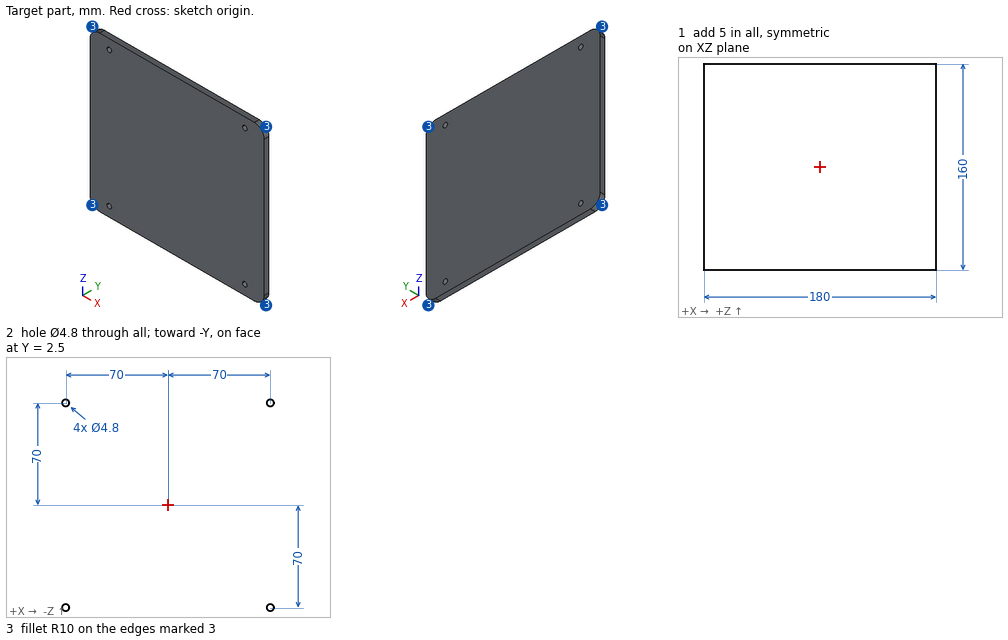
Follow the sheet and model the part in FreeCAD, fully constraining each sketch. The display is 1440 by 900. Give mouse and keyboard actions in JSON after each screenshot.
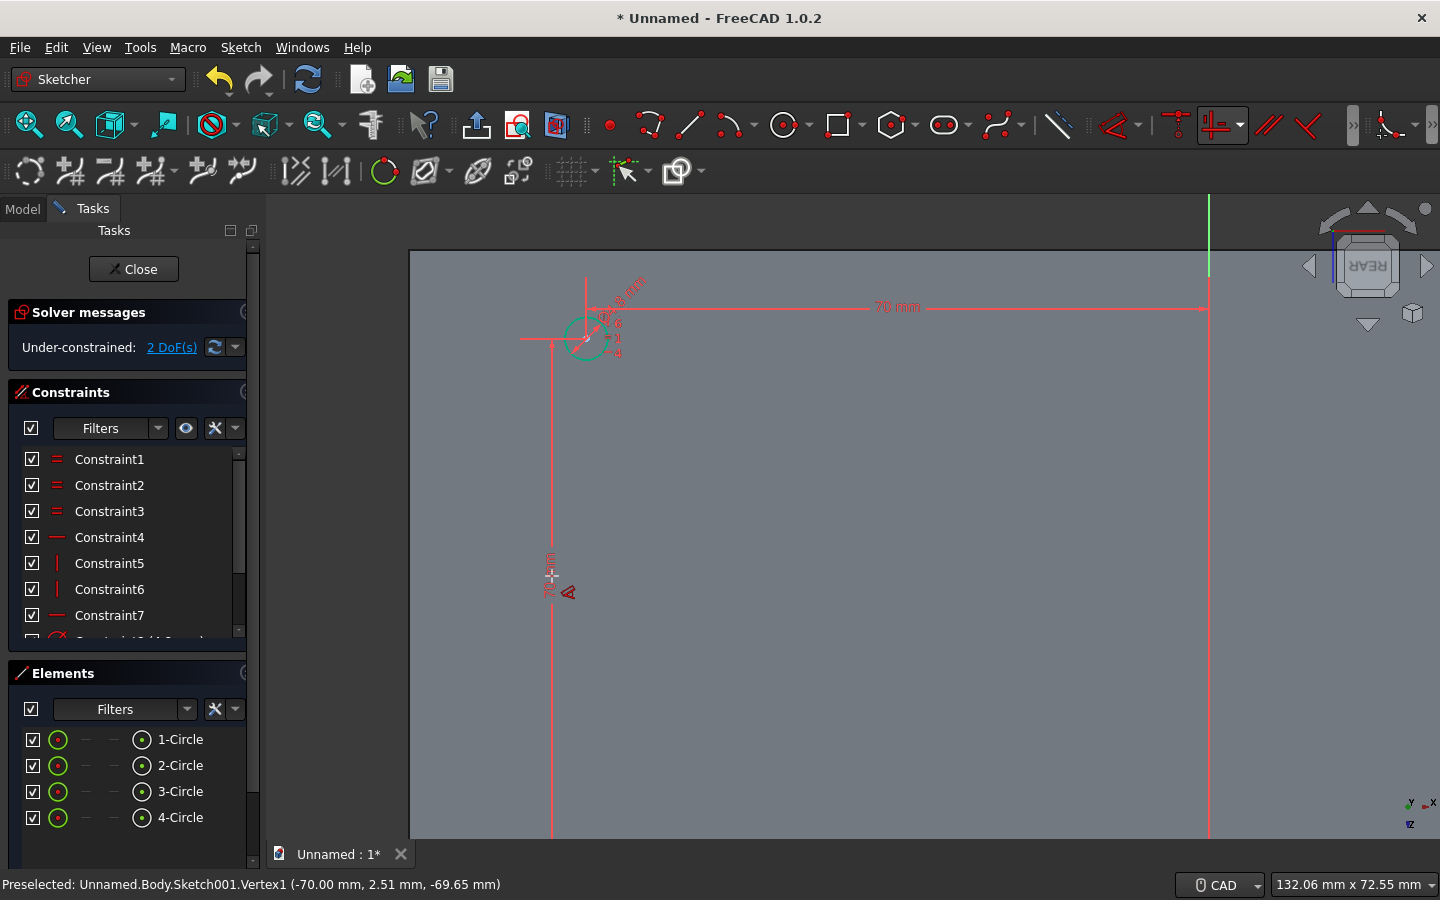
{"action": "scroll", "coordinate": [602, 325], "scroll_direction": "down", "scroll_amount": 6}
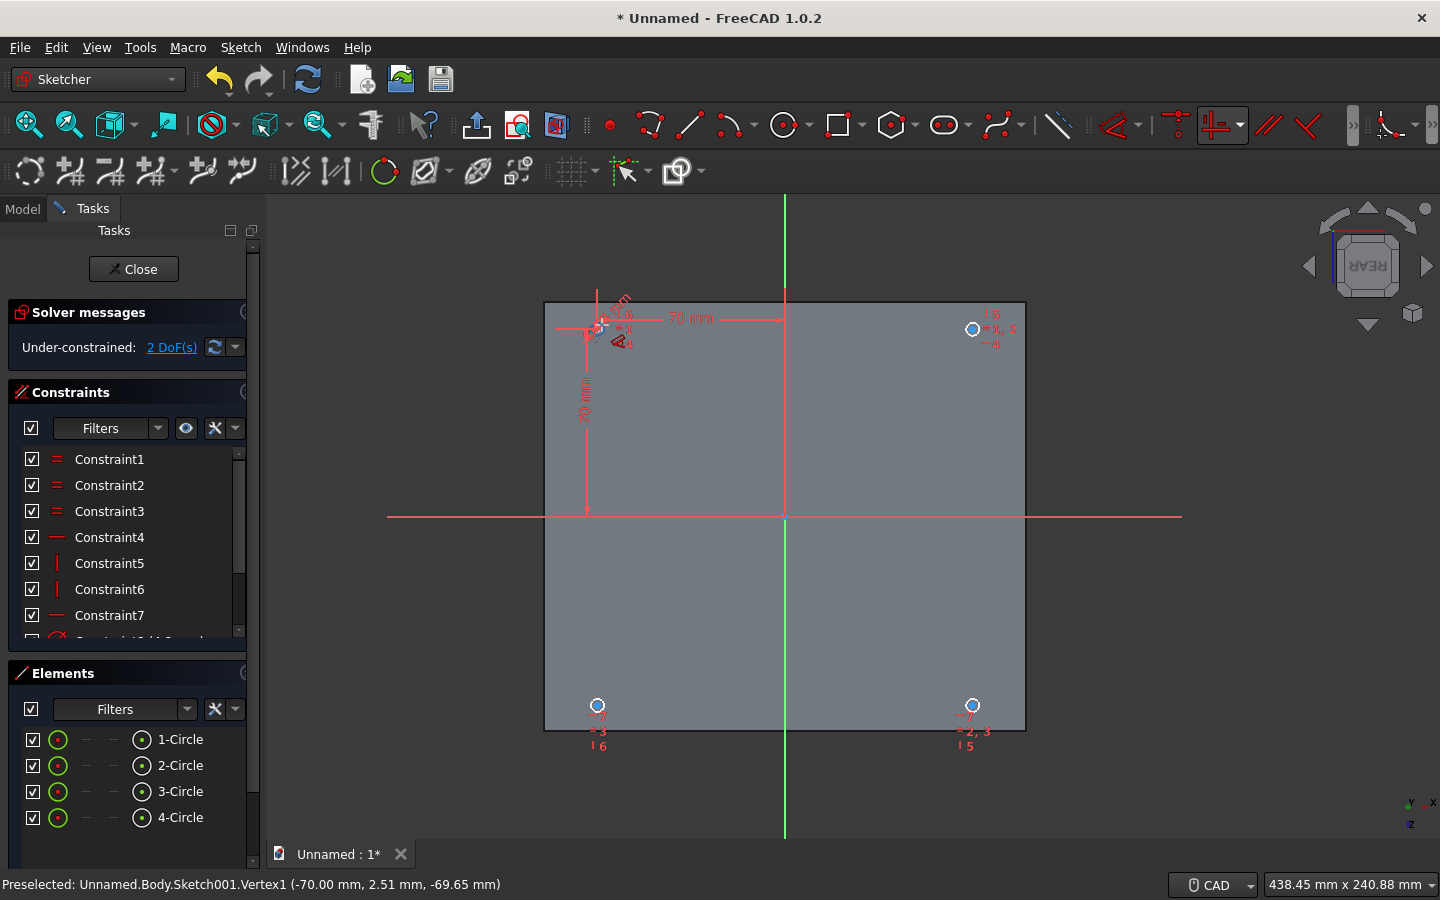
{"action": "left_click", "coordinate": [973, 329]}
{"action": "left_click", "coordinate": [879, 295]}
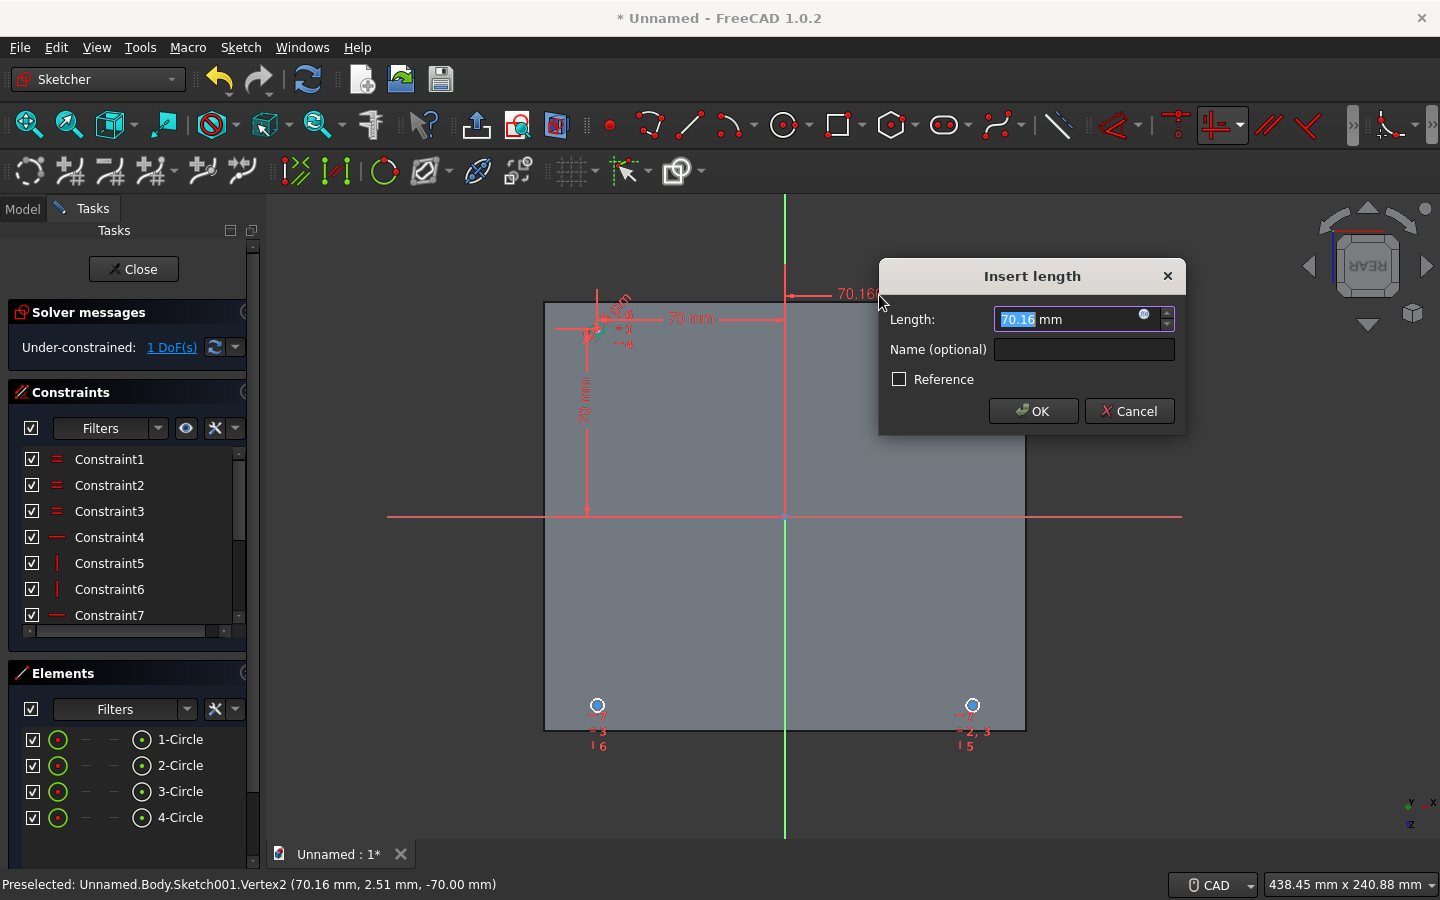
{"action": "type", "text": "70"}
{"action": "key", "text": "Return"}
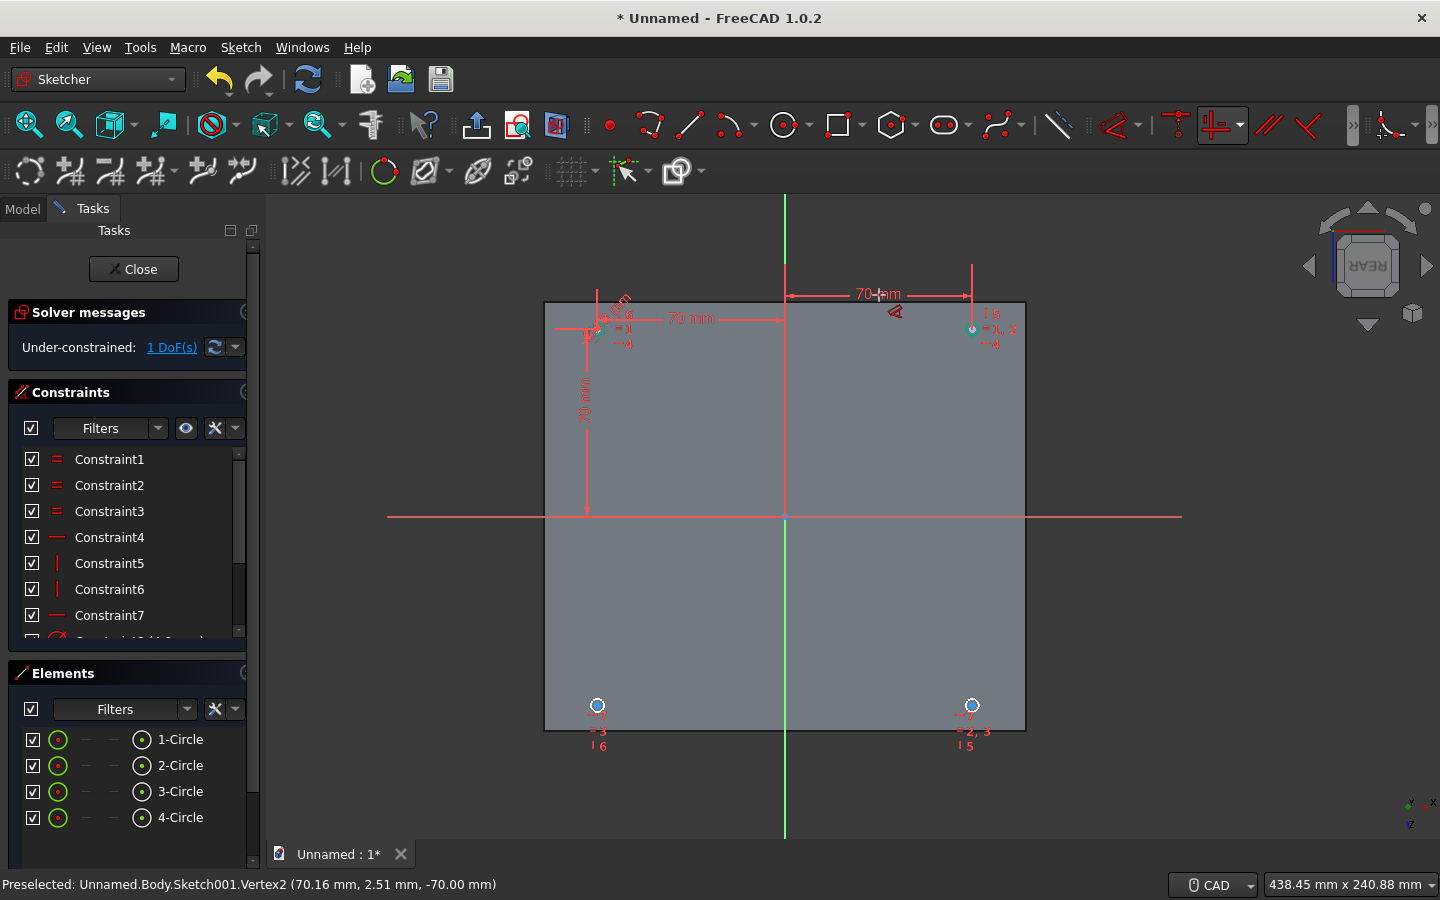
{"action": "left_click", "coordinate": [972, 705]}
{"action": "left_click", "coordinate": [1006, 611]}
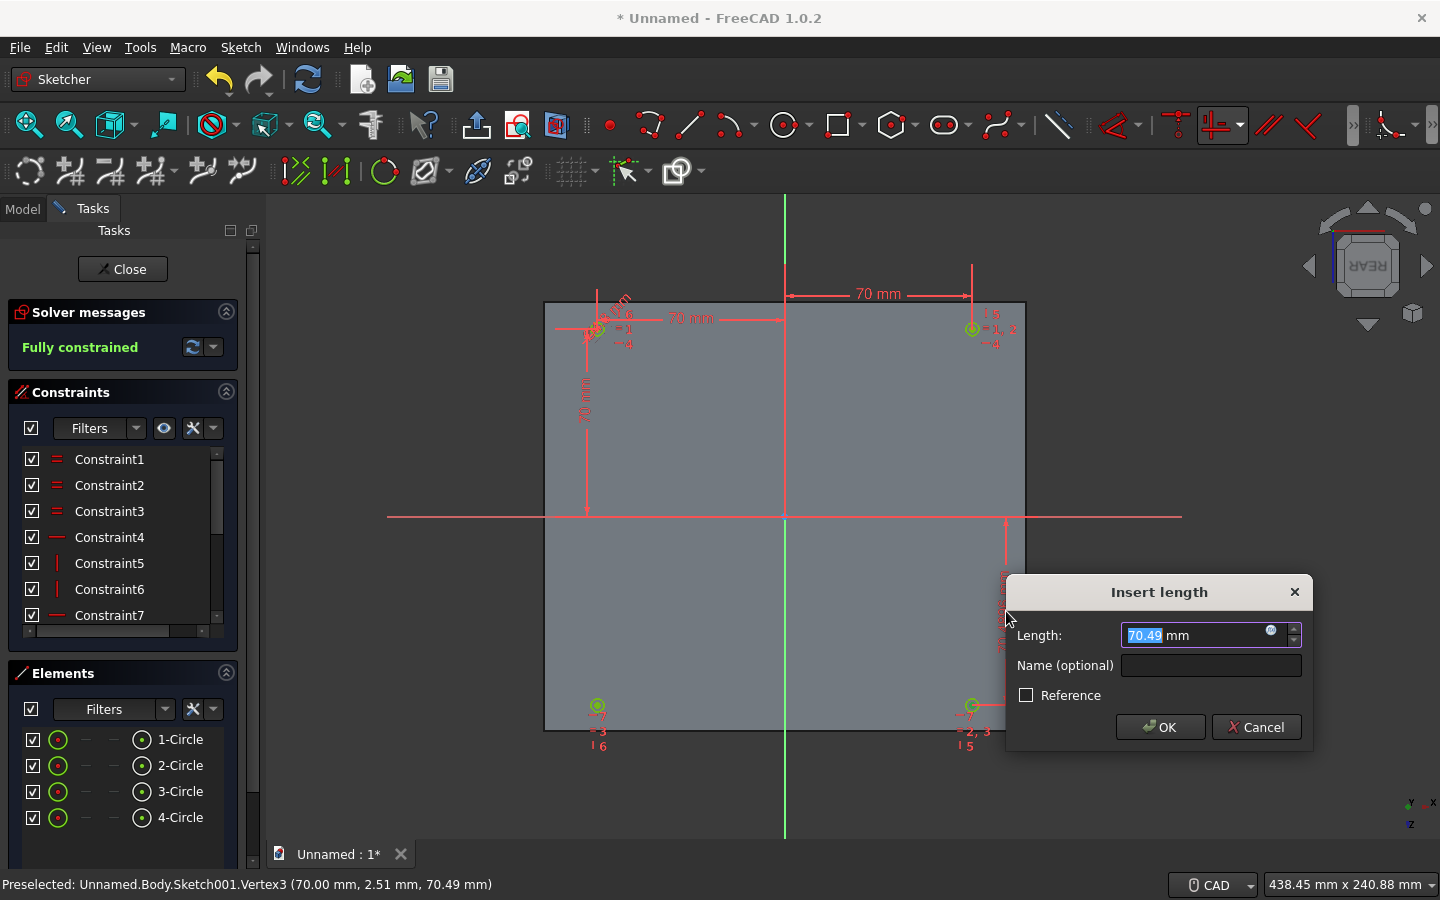
{"action": "type", "text": "70"}
{"action": "key", "text": "Return"}
{"action": "key", "text": "Escape"}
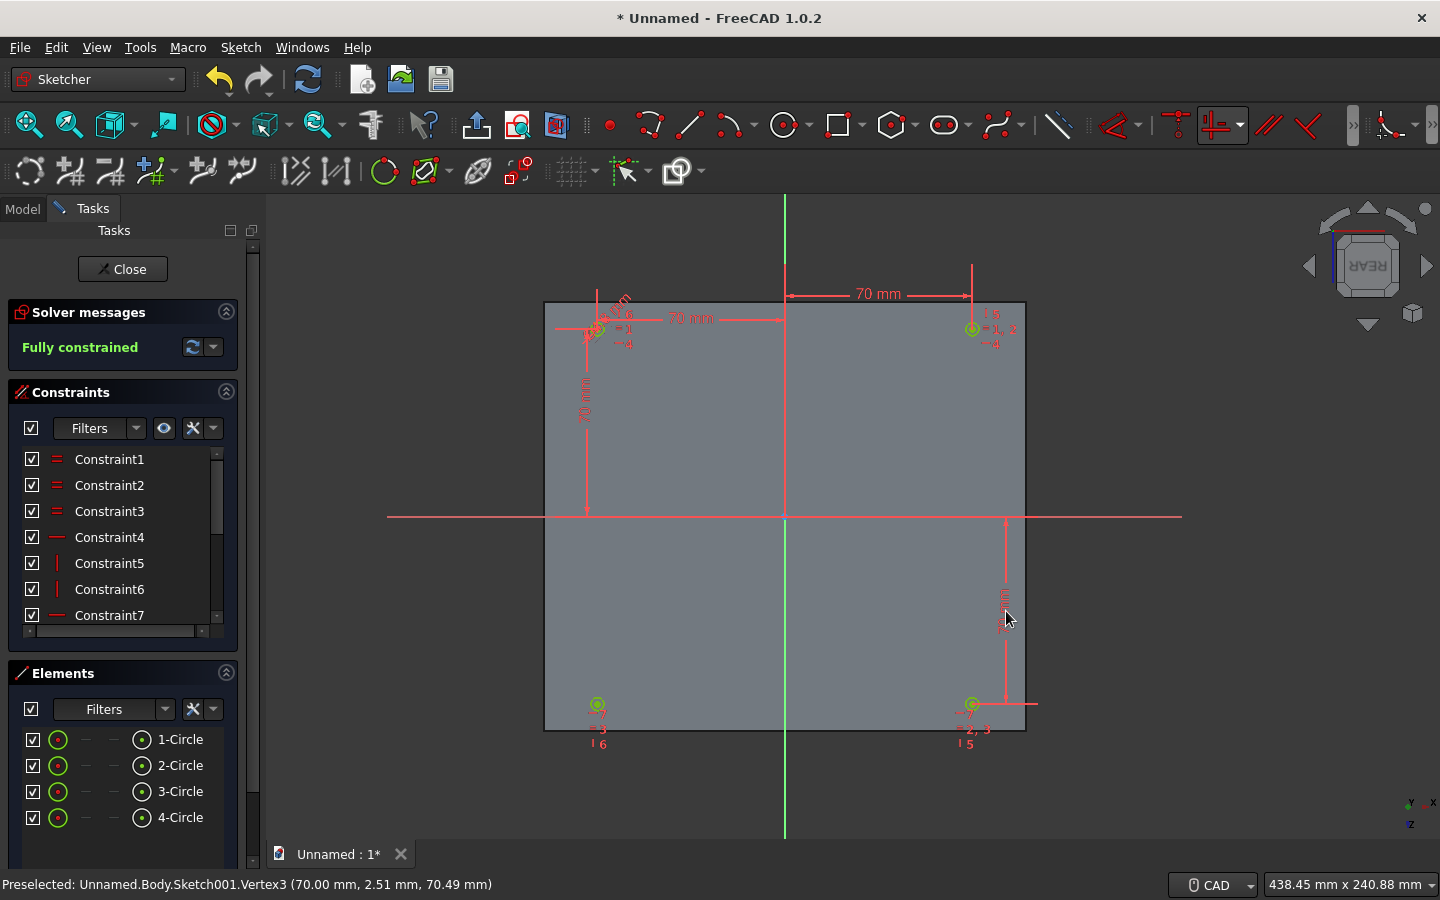
{"action": "left_click", "coordinate": [123, 269]}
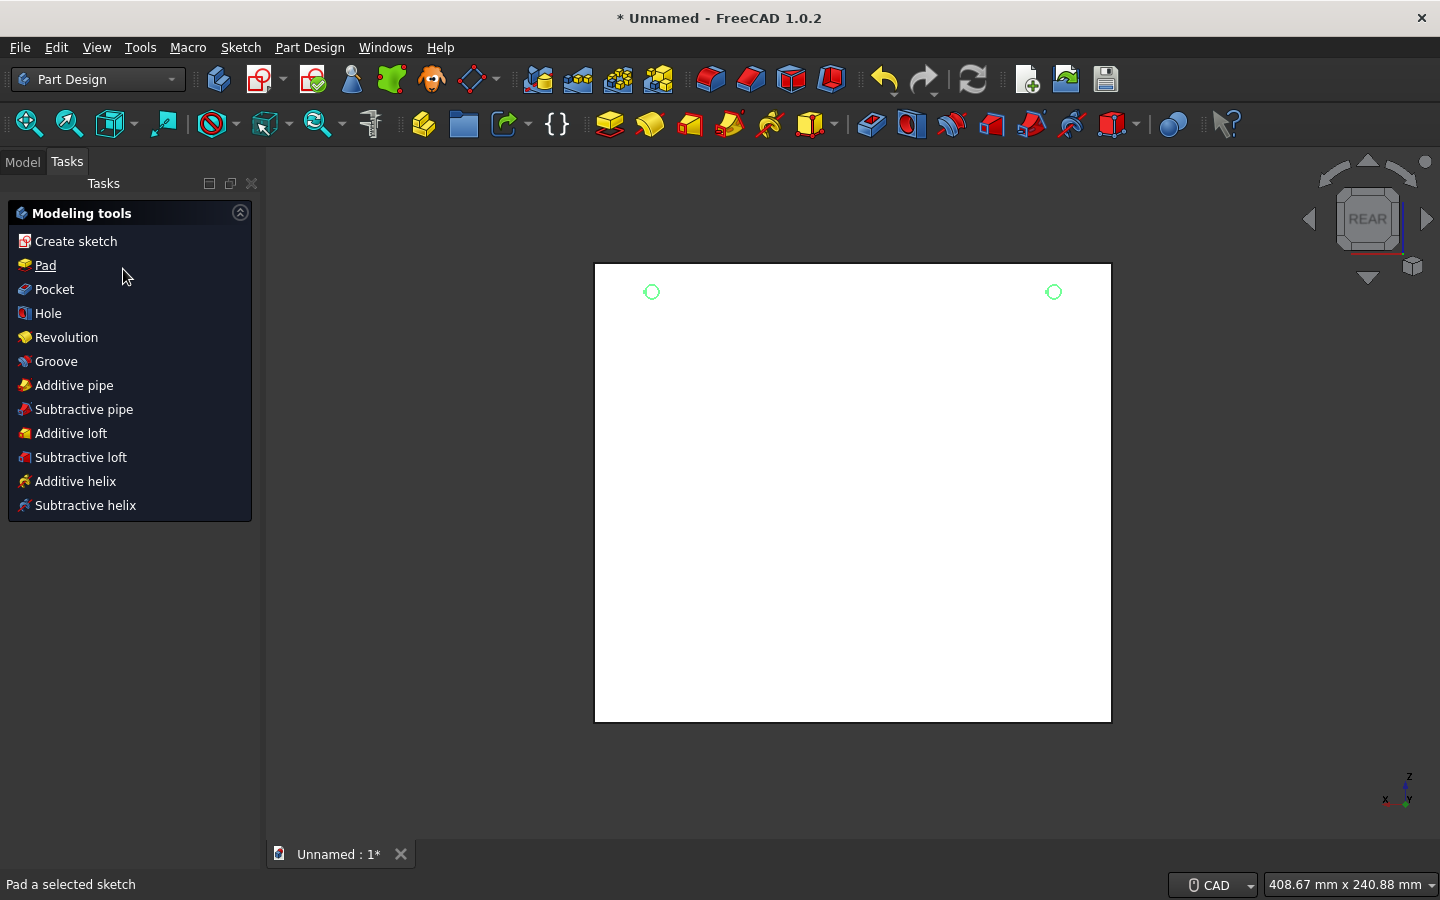
{"action": "left_click", "coordinate": [912, 124]}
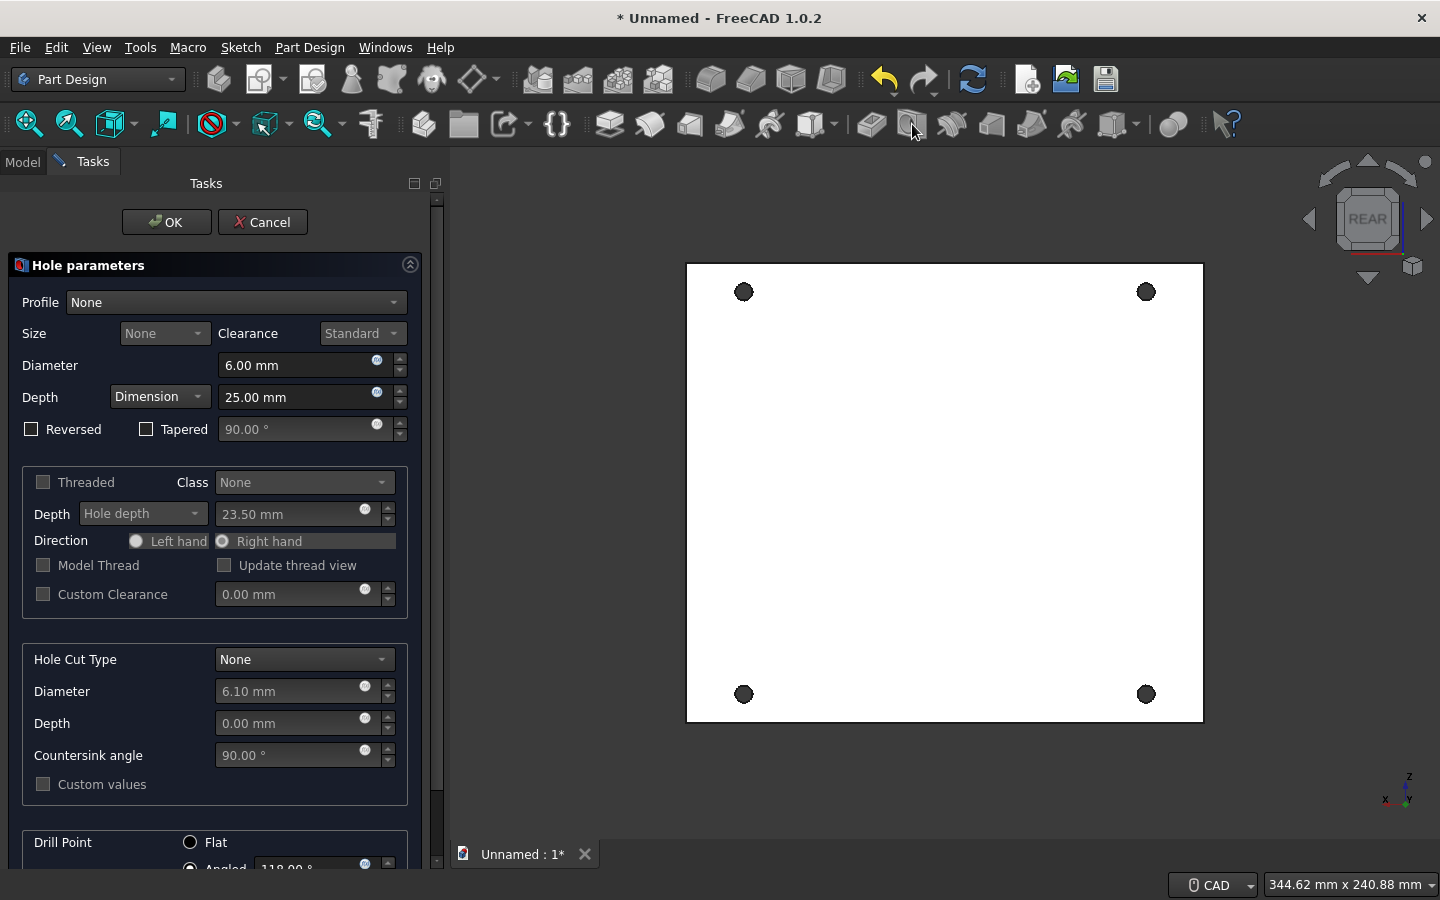
{"action": "triple_click", "coordinate": [305, 365]}